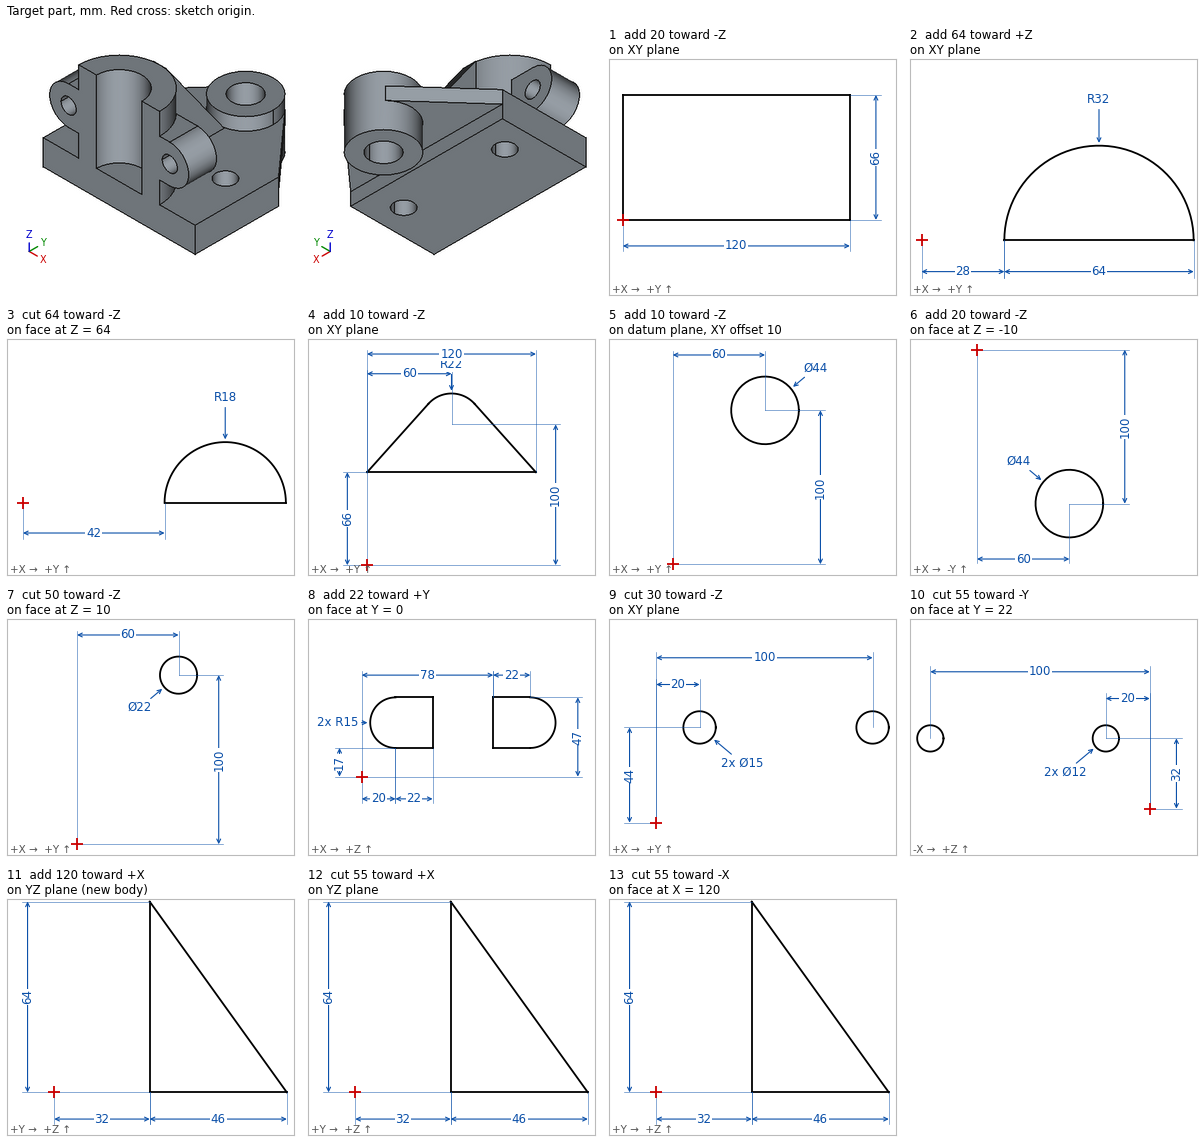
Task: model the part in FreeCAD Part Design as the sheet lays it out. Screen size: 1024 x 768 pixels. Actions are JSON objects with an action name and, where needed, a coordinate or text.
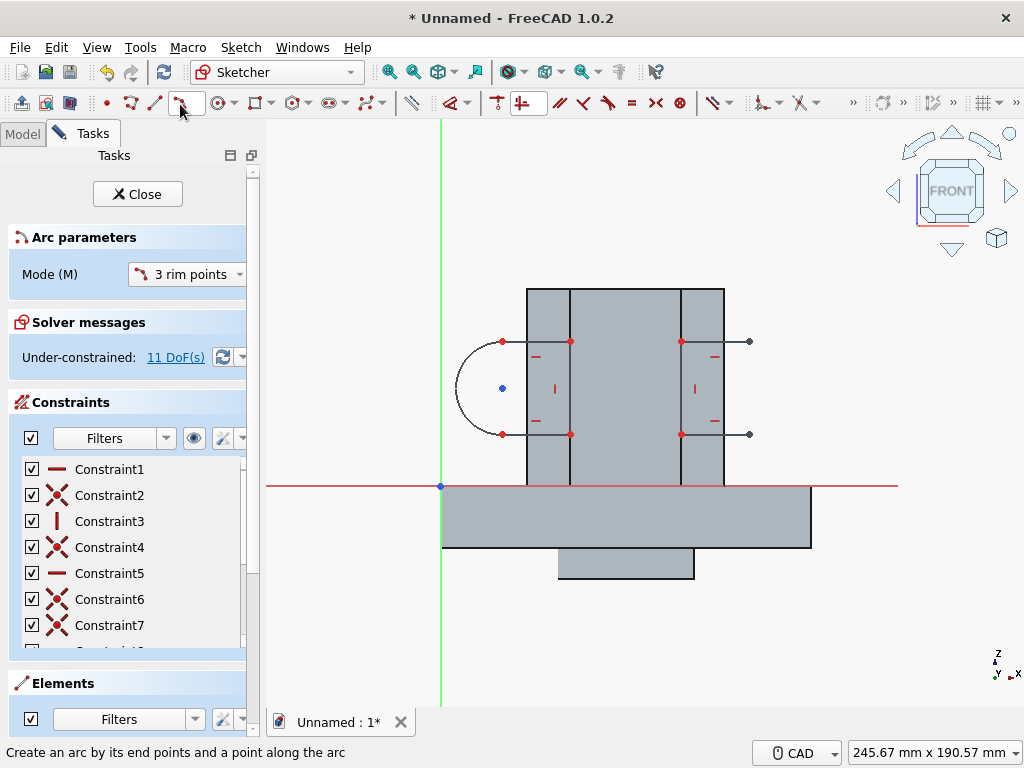
{"action": "left_click", "coordinate": [749, 435]}
{"action": "left_click", "coordinate": [749, 342]}
{"action": "left_click", "coordinate": [795, 387]}
{"action": "key", "text": "Escape"}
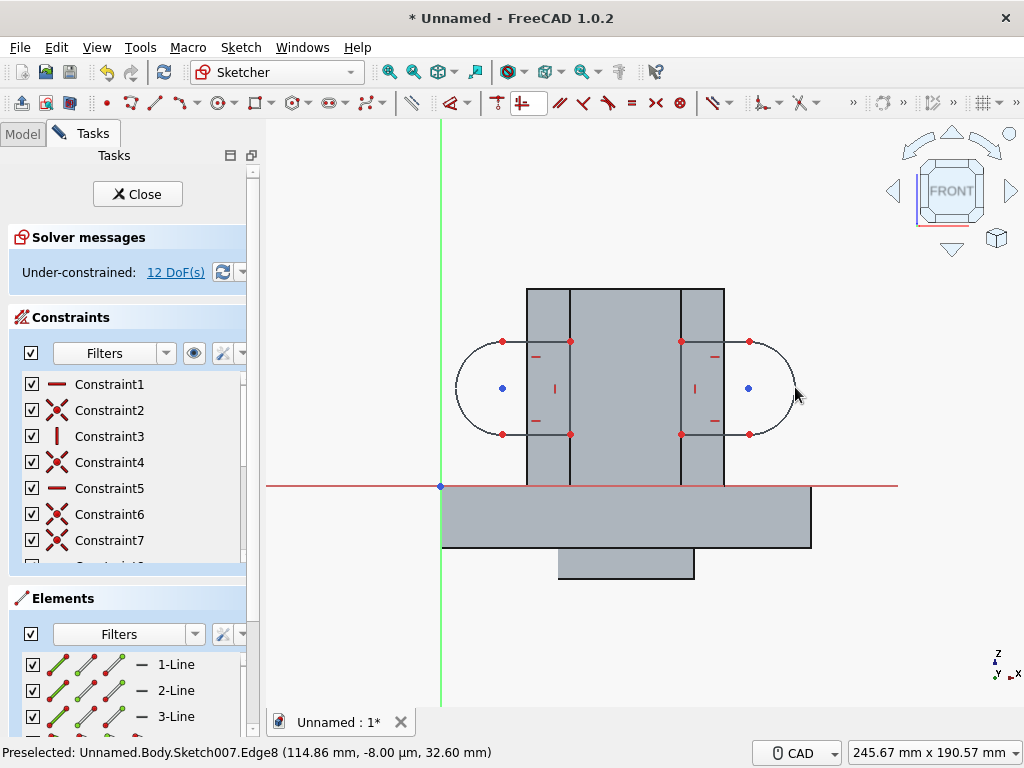
{"action": "left_click", "coordinate": [522, 435]}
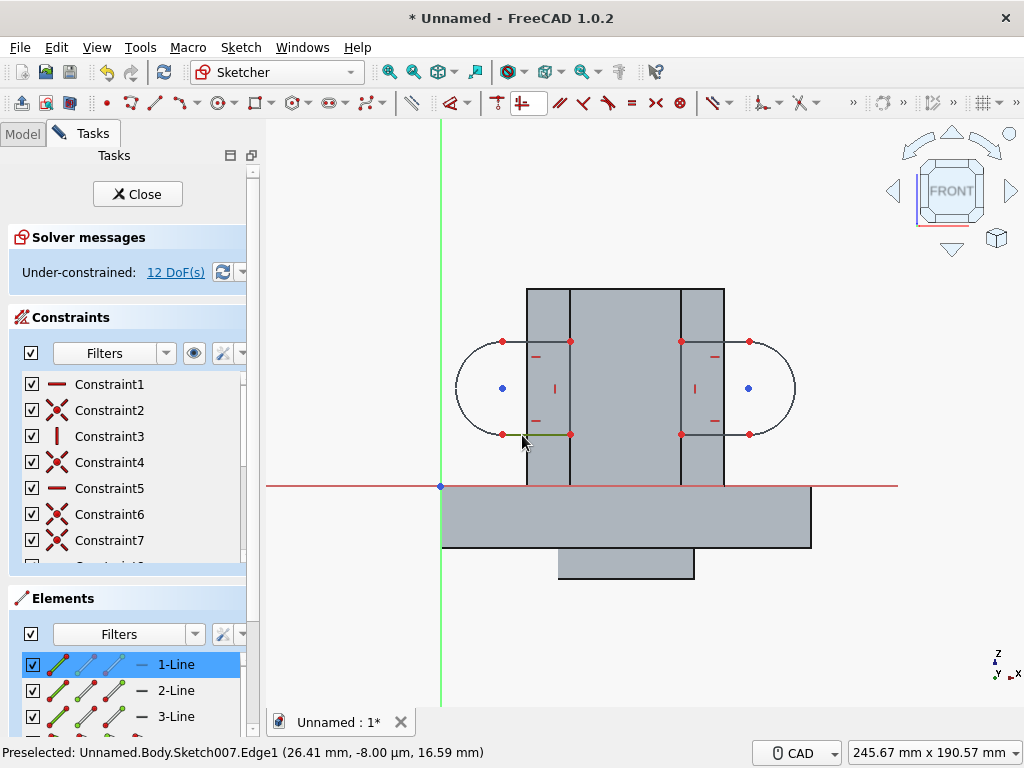
{"action": "left_click", "coordinate": [465, 361]}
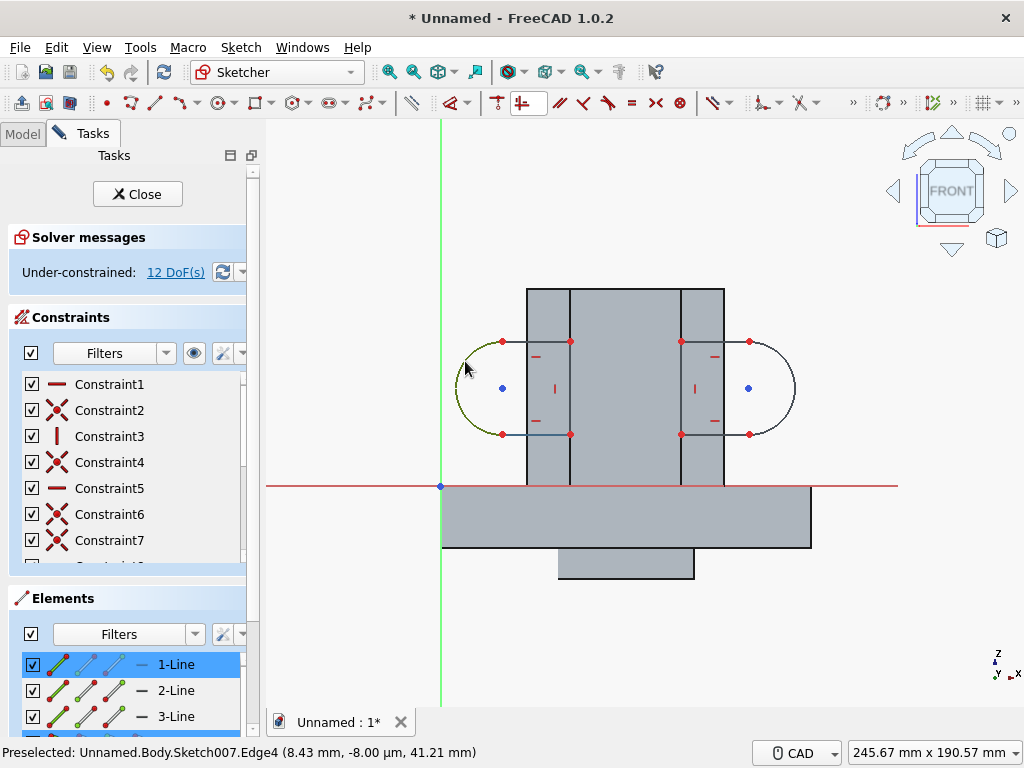
{"action": "left_click", "coordinate": [608, 104]}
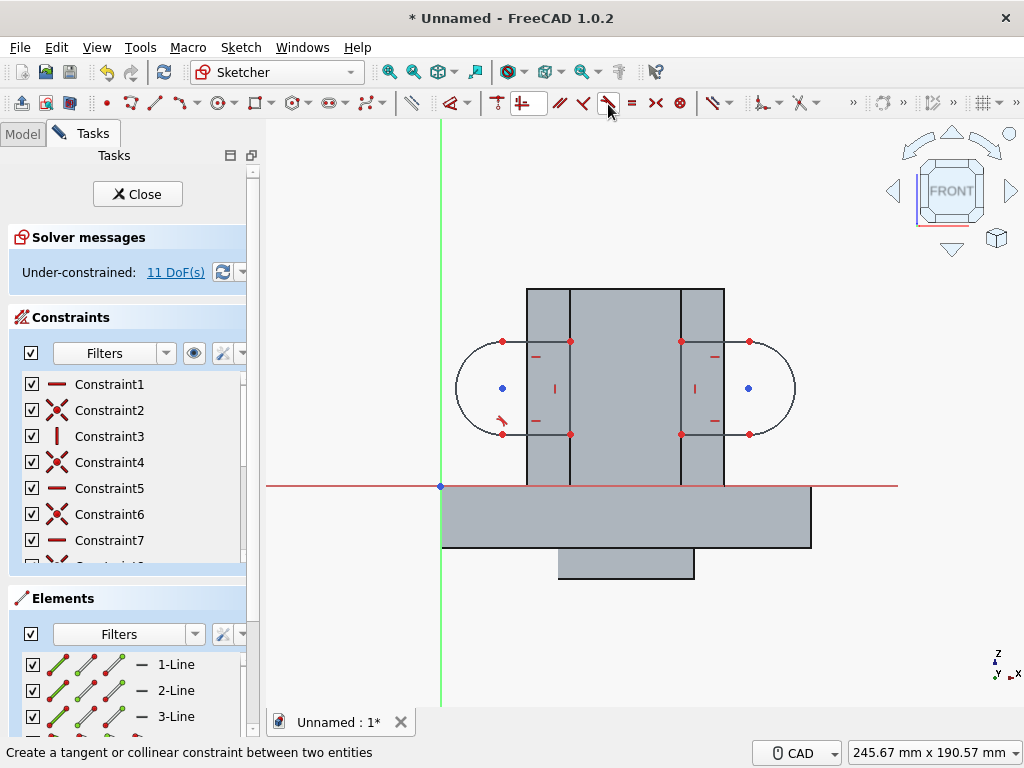
{"action": "left_click", "coordinate": [550, 342]}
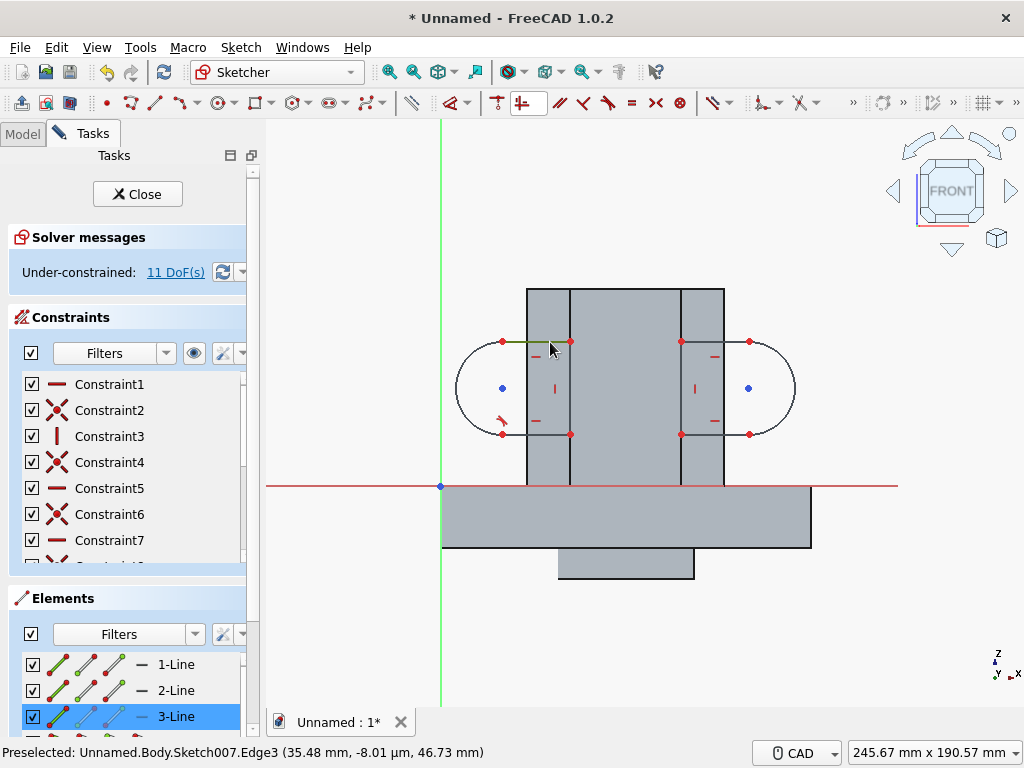
{"action": "left_click", "coordinate": [465, 361]}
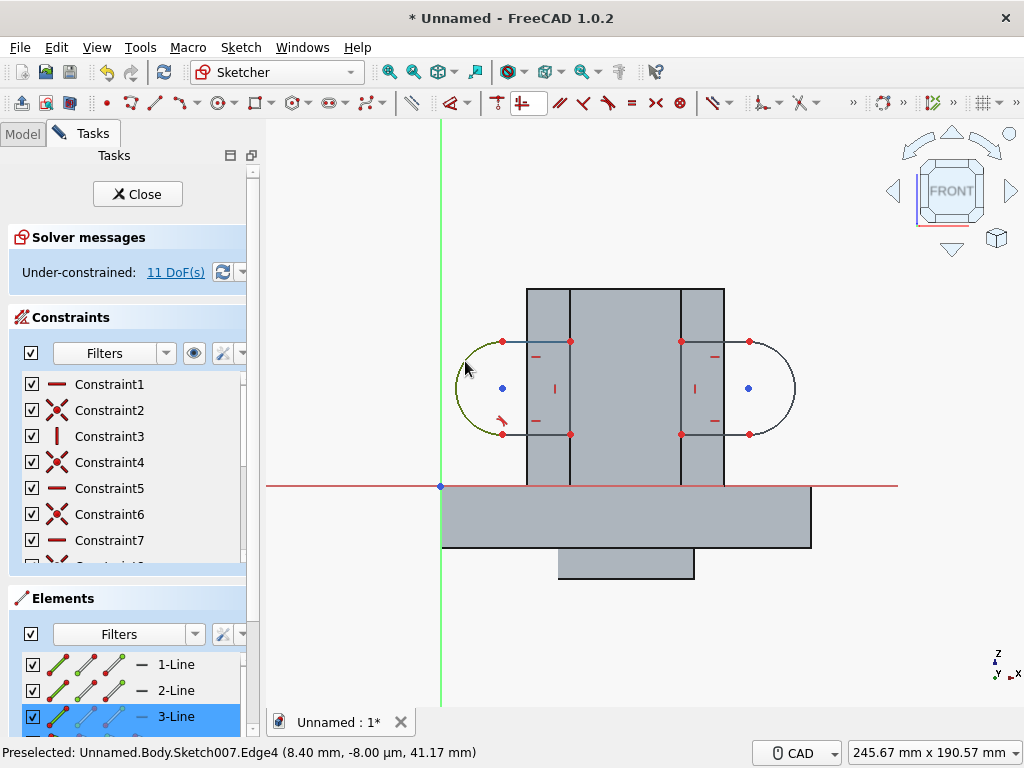
{"action": "left_click", "coordinate": [608, 104]}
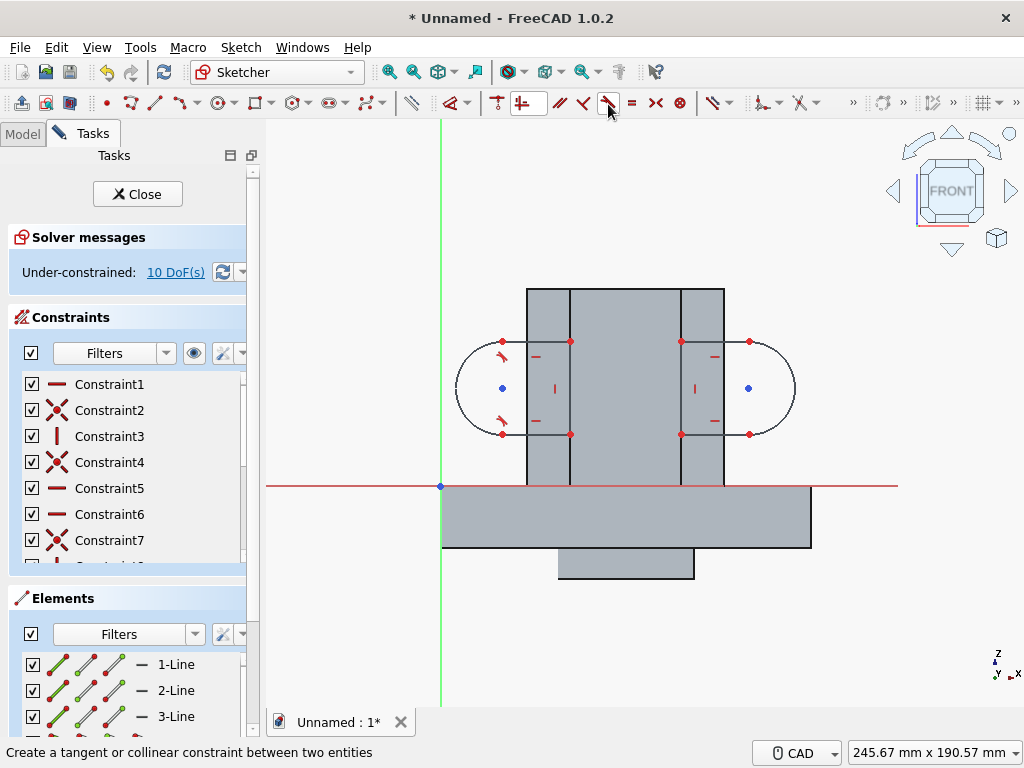
{"action": "left_click", "coordinate": [729, 342]}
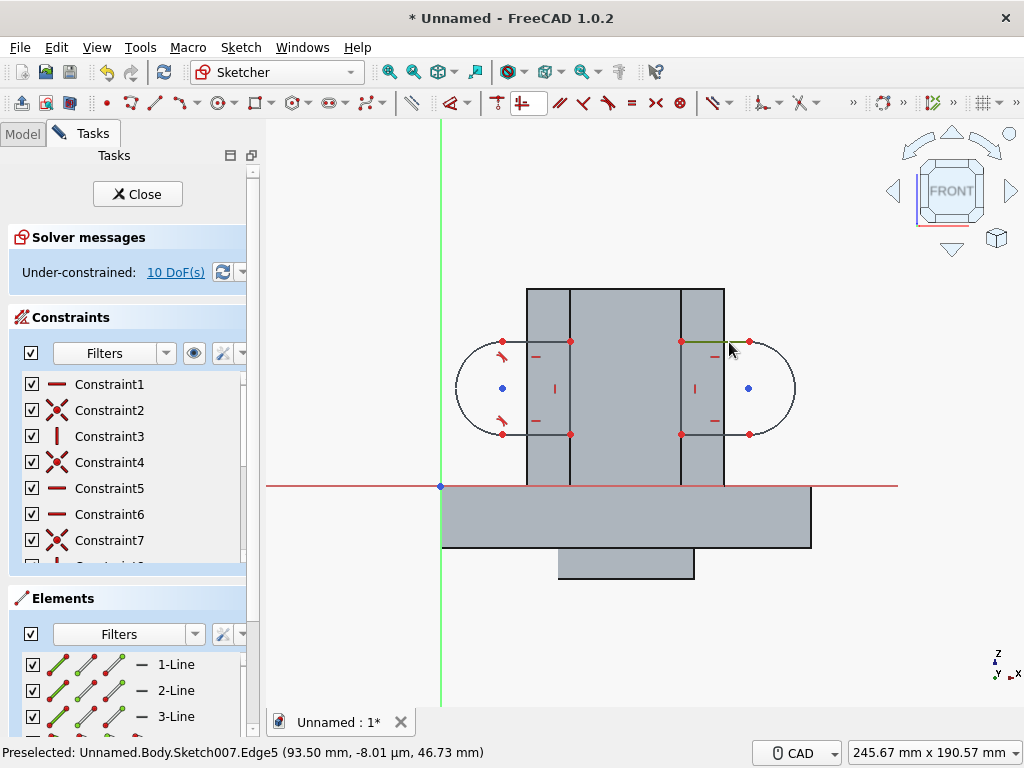
{"action": "left_click", "coordinate": [786, 416]}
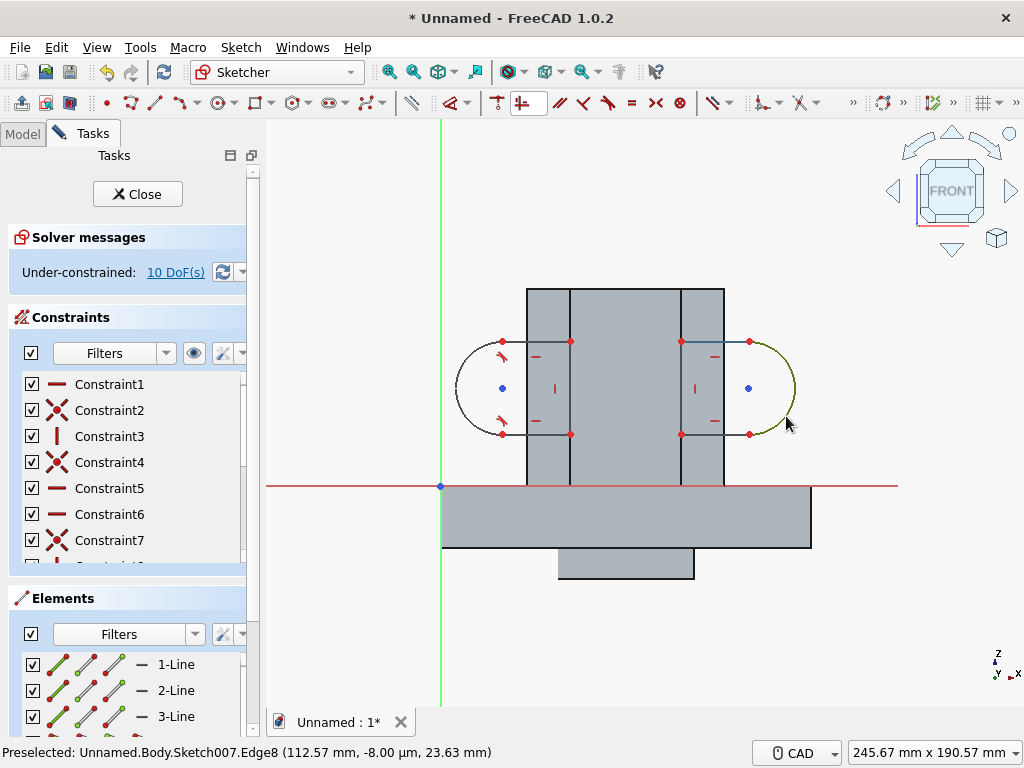
{"action": "left_click", "coordinate": [608, 104]}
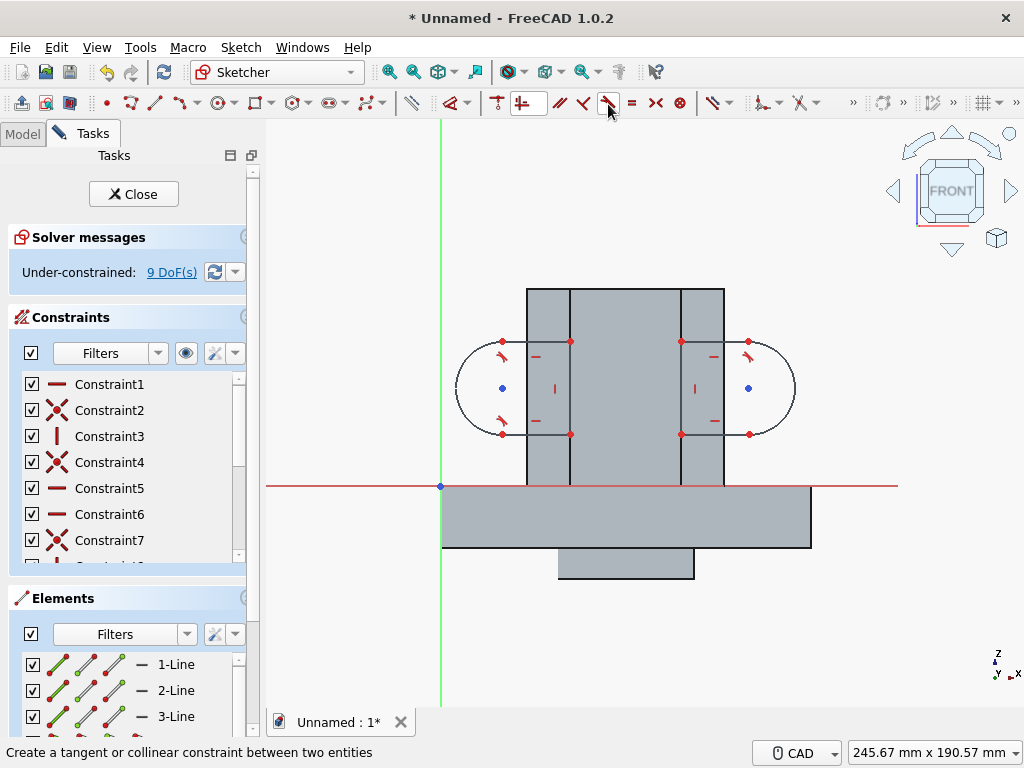
{"action": "left_click", "coordinate": [701, 435]}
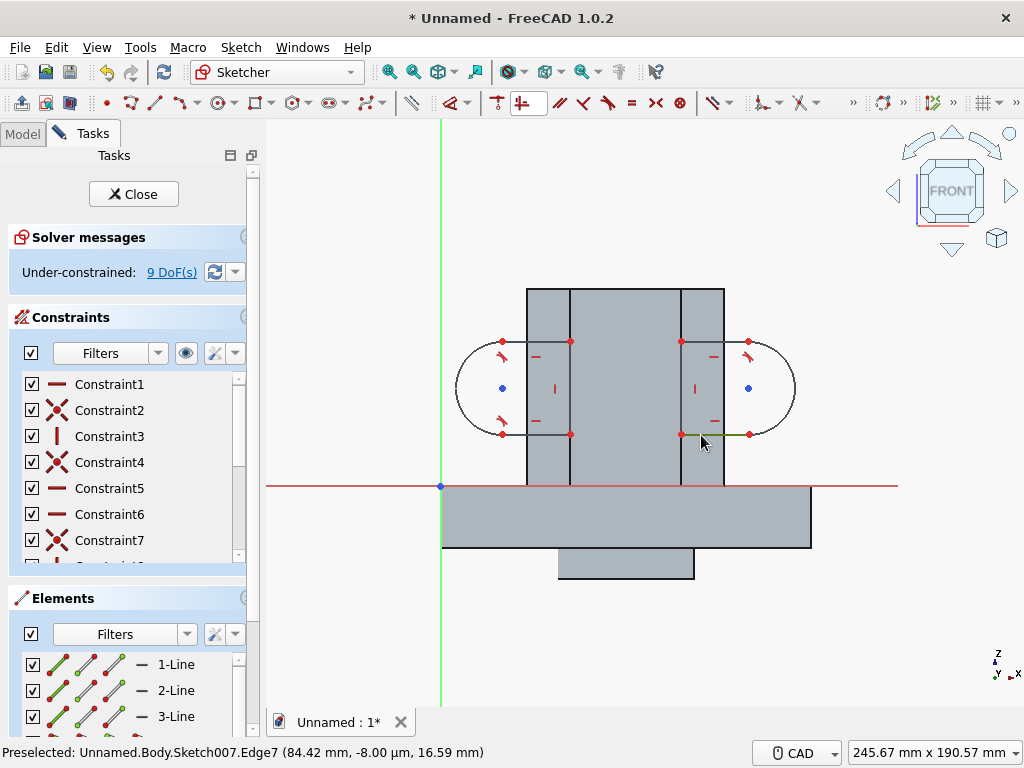
{"action": "left_click", "coordinate": [786, 416]}